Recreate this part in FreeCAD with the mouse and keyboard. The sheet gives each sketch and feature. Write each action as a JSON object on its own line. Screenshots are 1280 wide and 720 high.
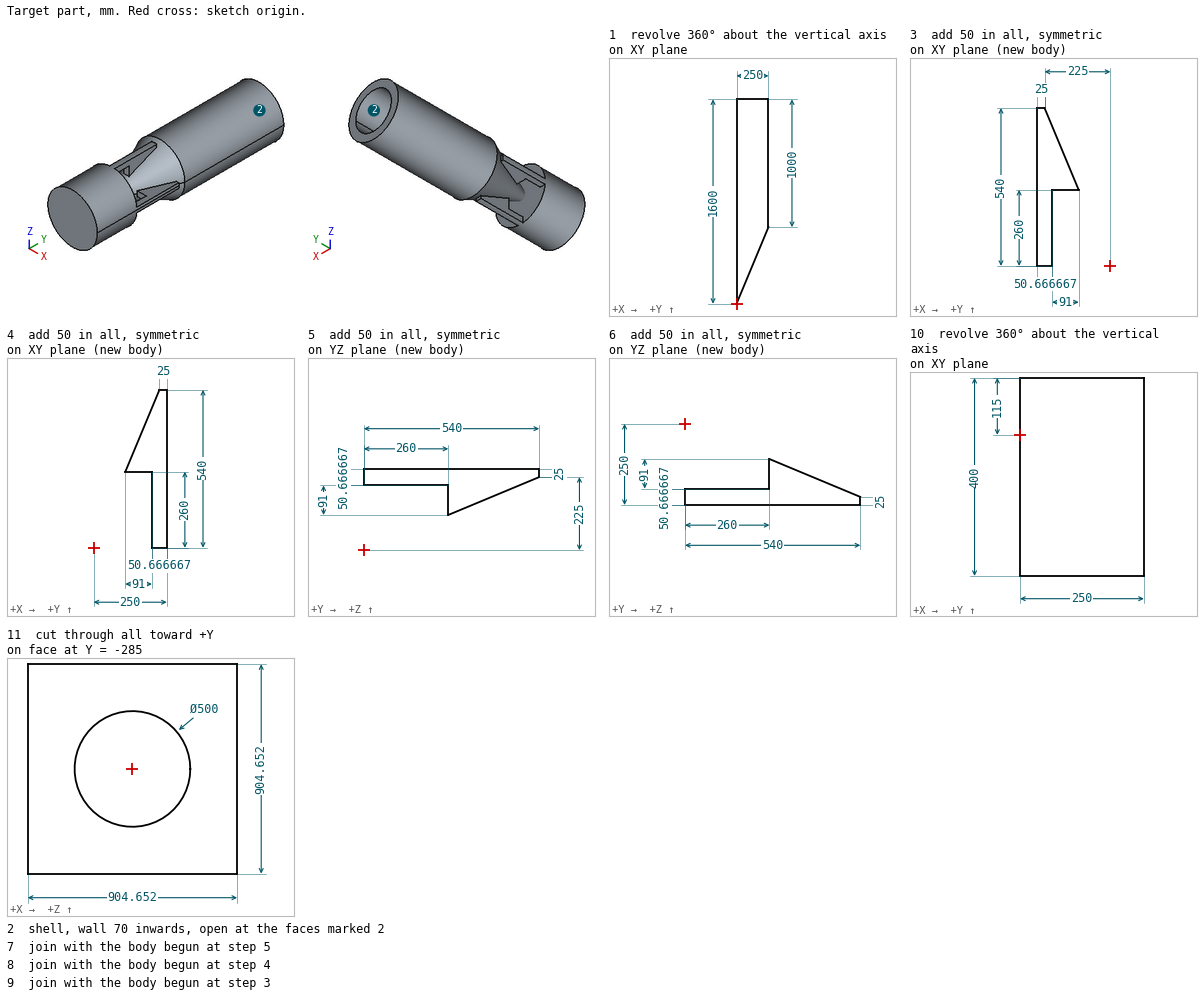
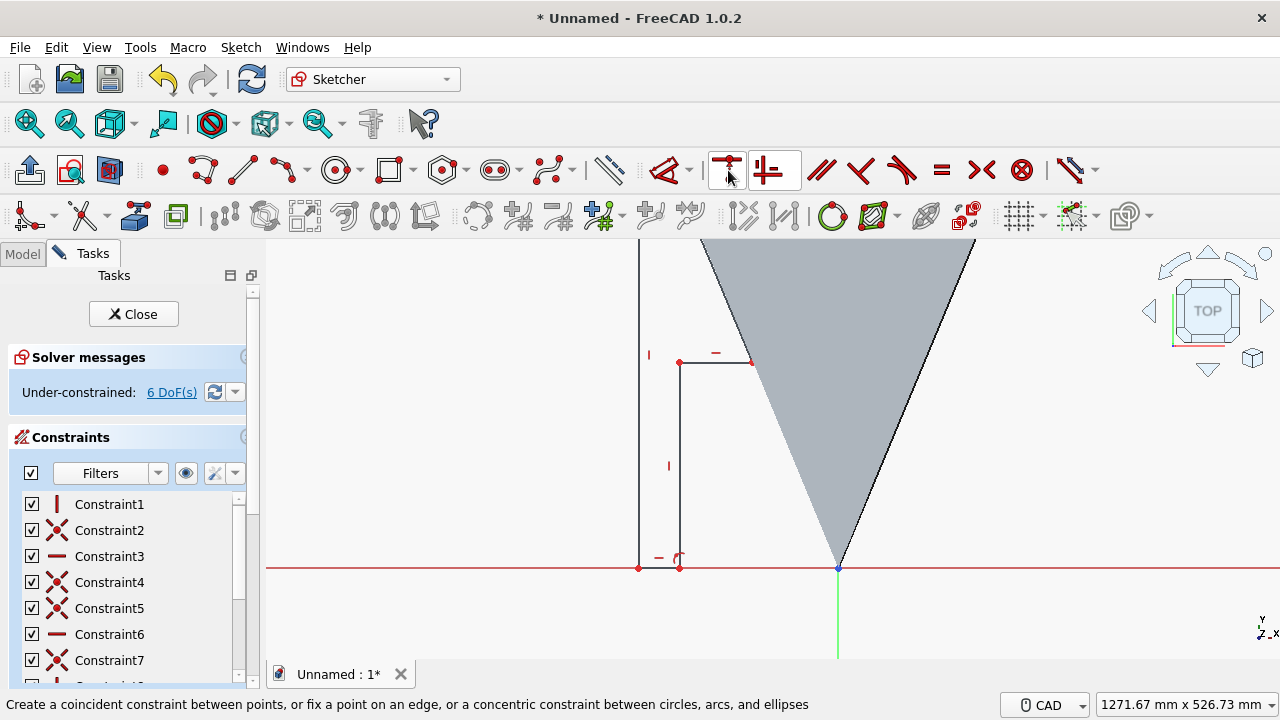
{"action": "left_click", "coordinate": [664, 170]}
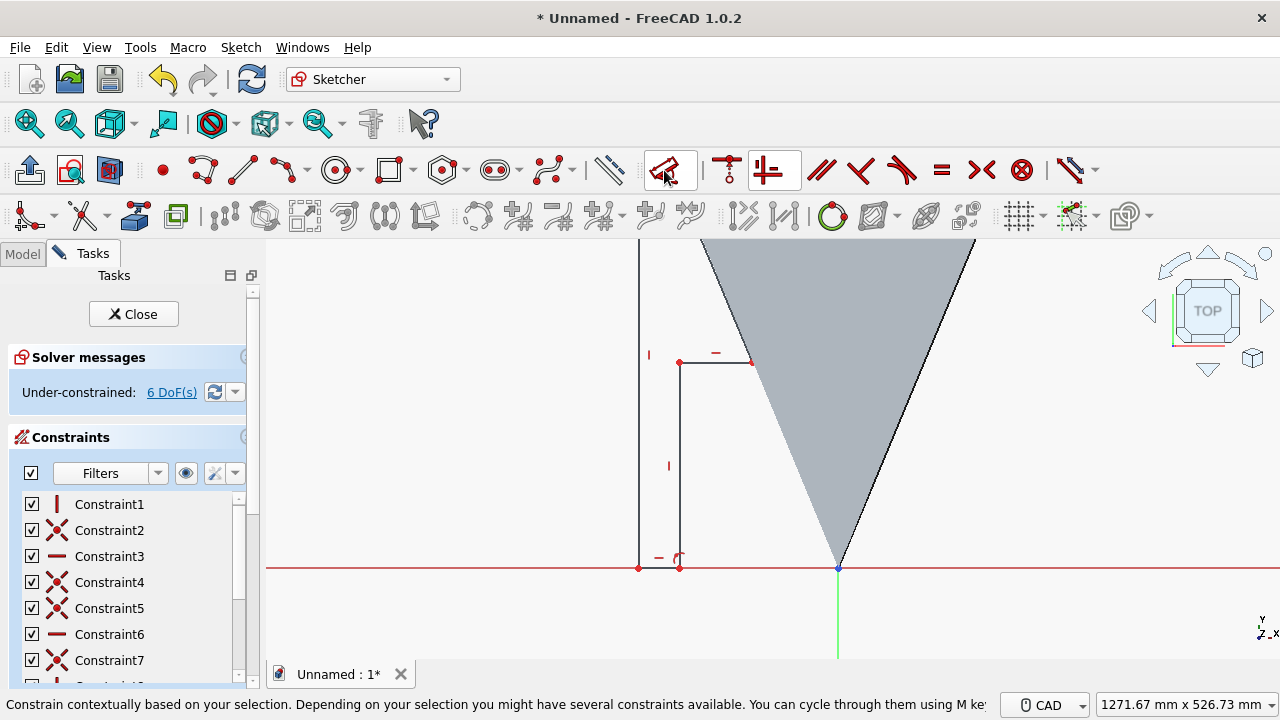
{"action": "left_click", "coordinate": [702, 363]}
{"action": "left_click", "coordinate": [716, 397]}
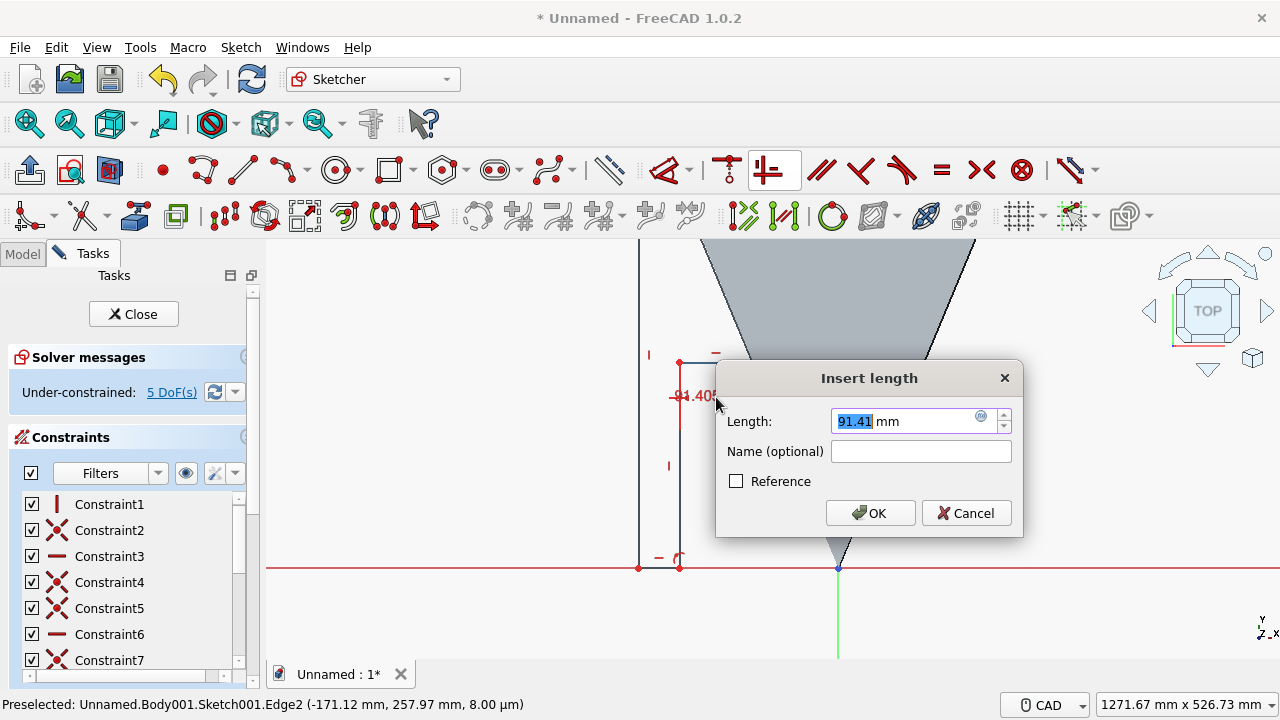
{"action": "type", "text": "91"}
{"action": "key", "text": "Return"}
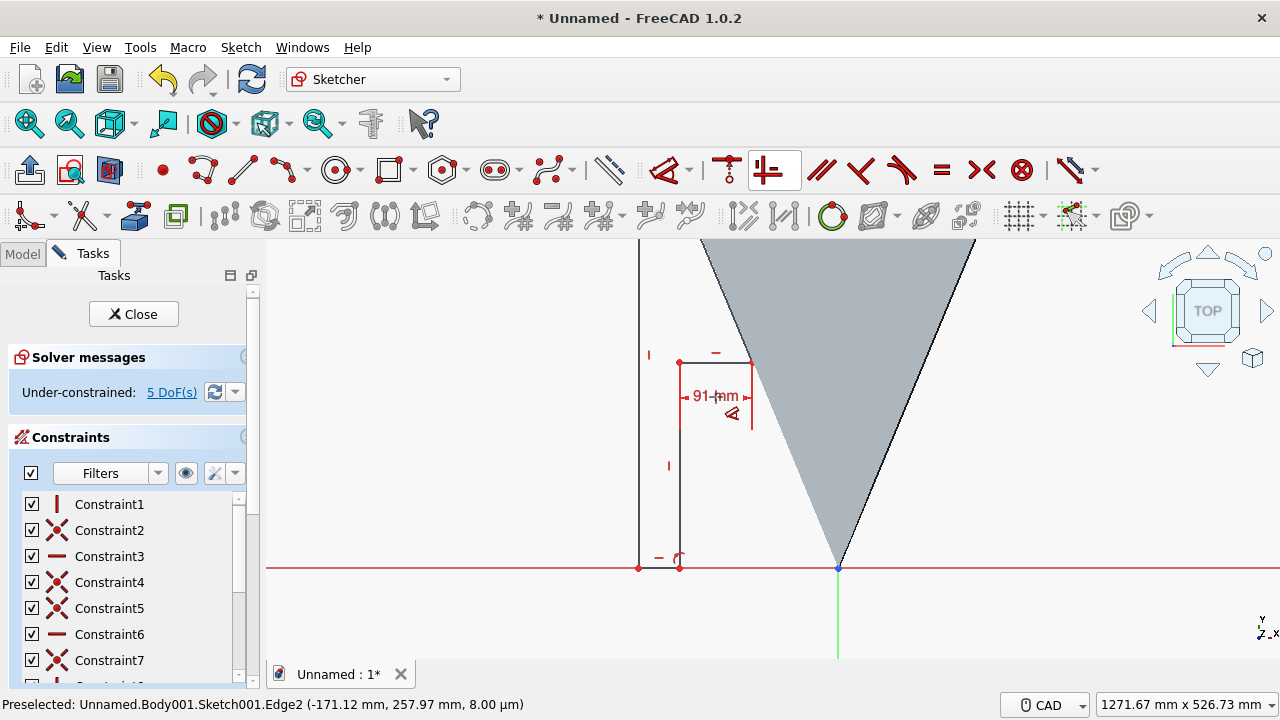
{"action": "scroll", "coordinate": [663, 566], "scroll_direction": "down", "scroll_amount": 3}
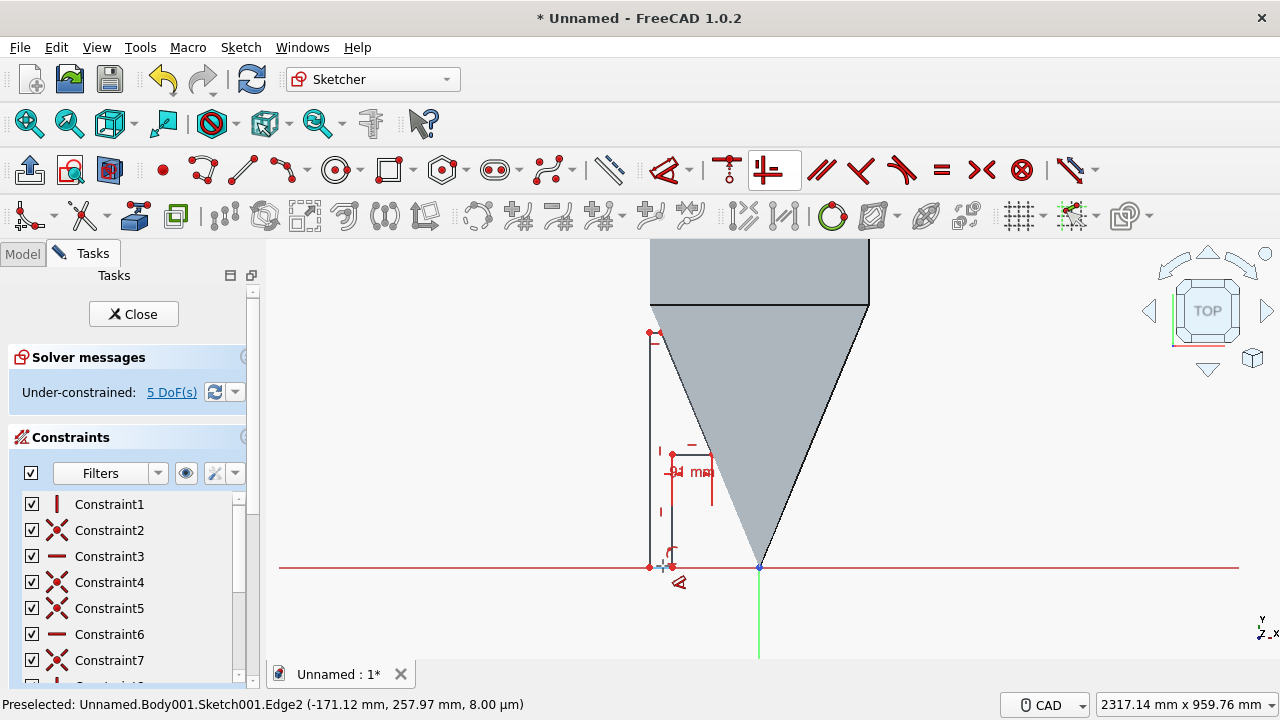
{"action": "scroll", "coordinate": [656, 333], "scroll_direction": "up", "scroll_amount": 7}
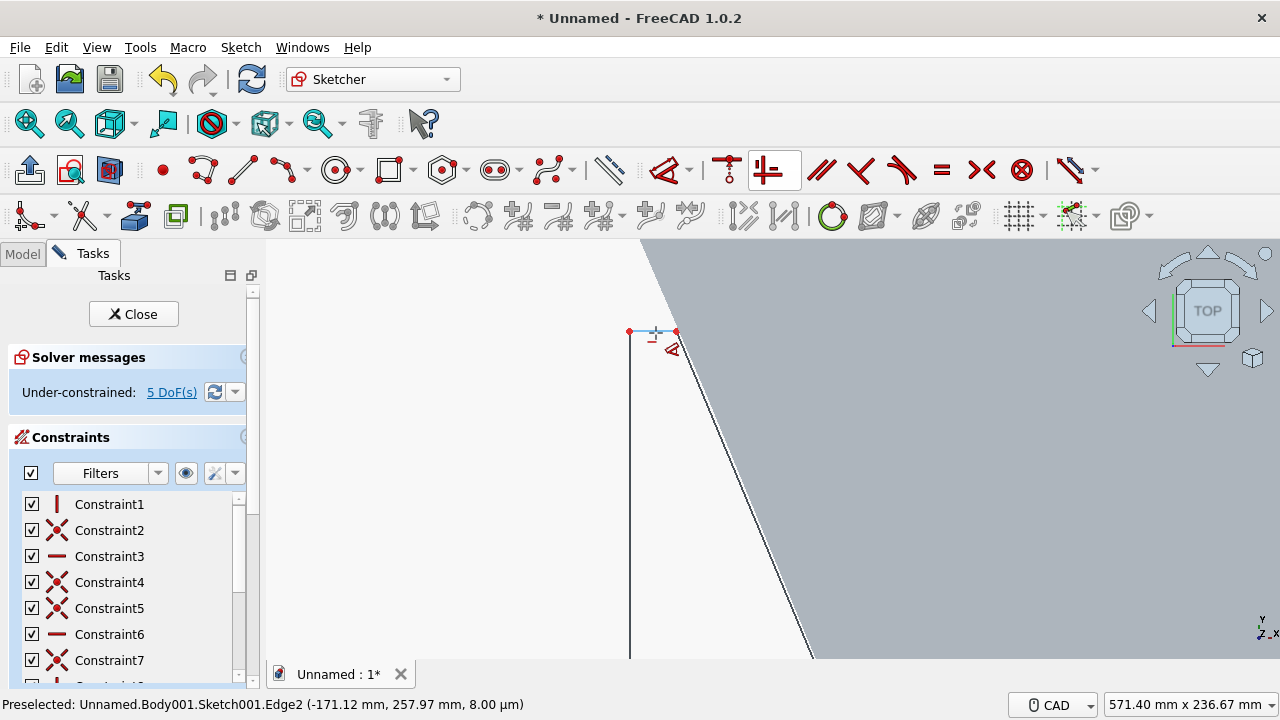
{"action": "left_click", "coordinate": [653, 331]}
{"action": "left_click", "coordinate": [653, 297]}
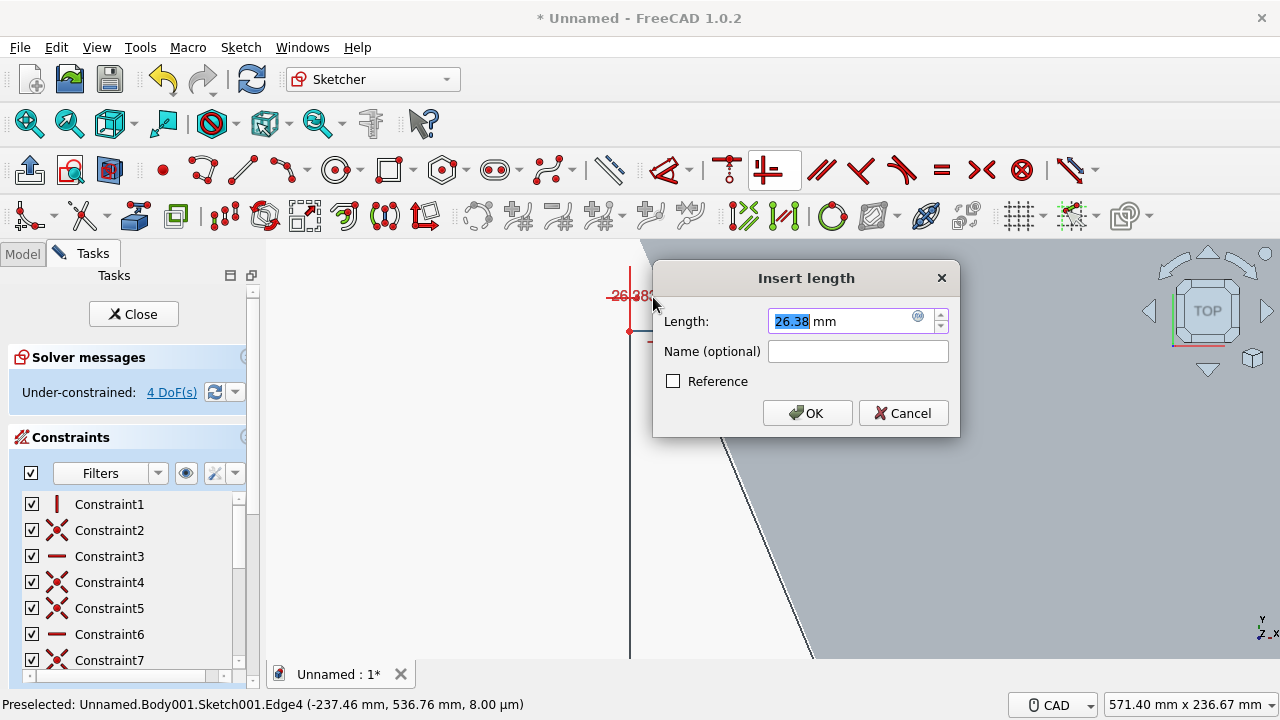
{"action": "type", "text": "25"}
{"action": "key", "text": "Return"}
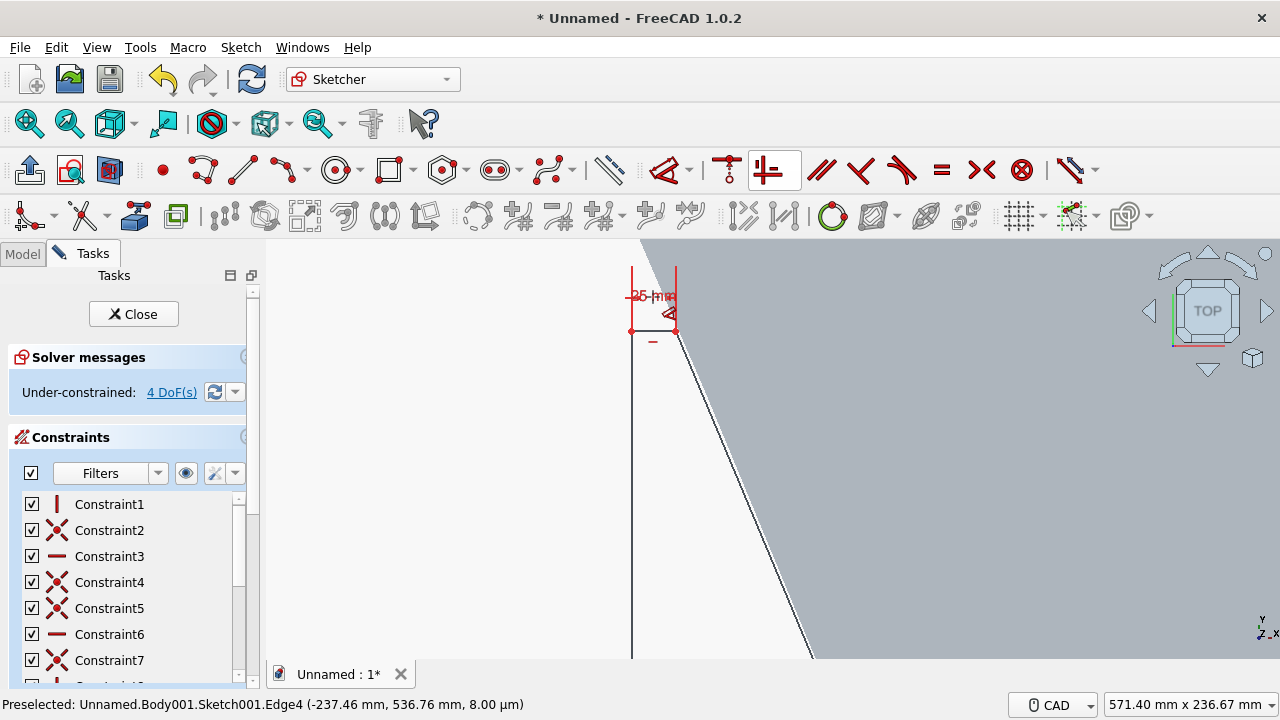
{"action": "scroll", "coordinate": [656, 333], "scroll_direction": "down", "scroll_amount": 7}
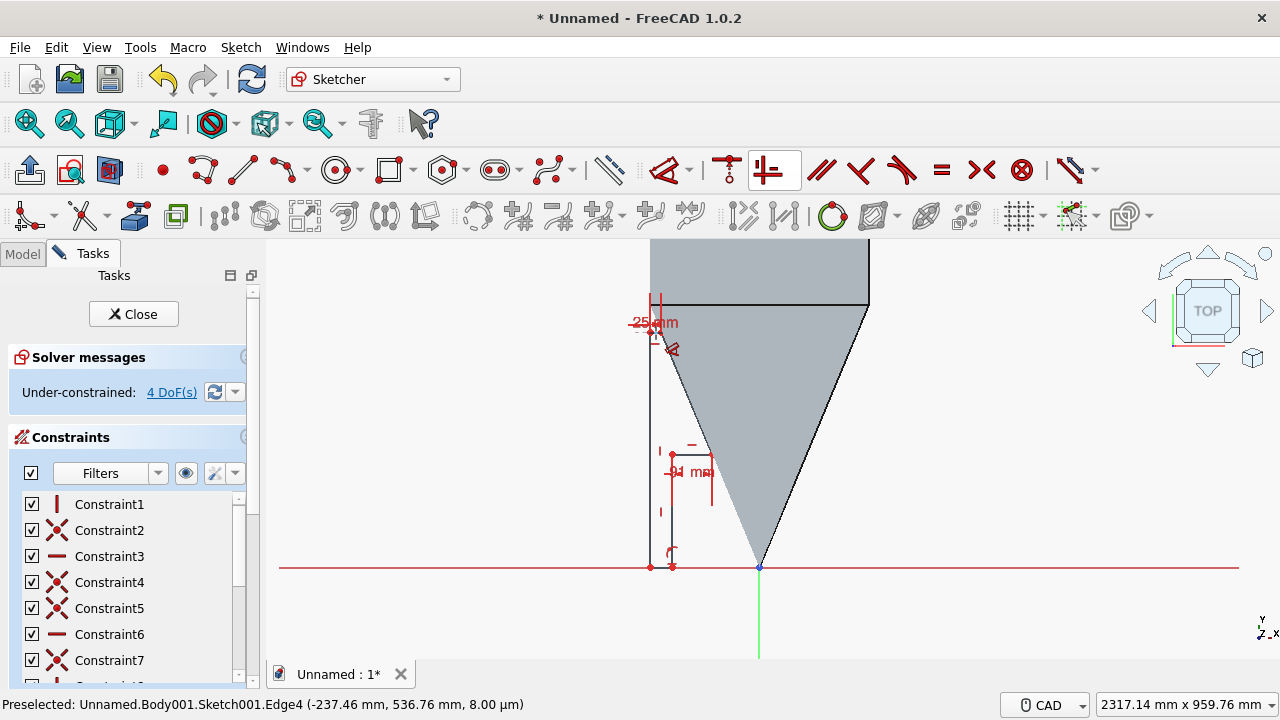
{"action": "left_click", "coordinate": [672, 534]}
{"action": "left_click", "coordinate": [706, 511]}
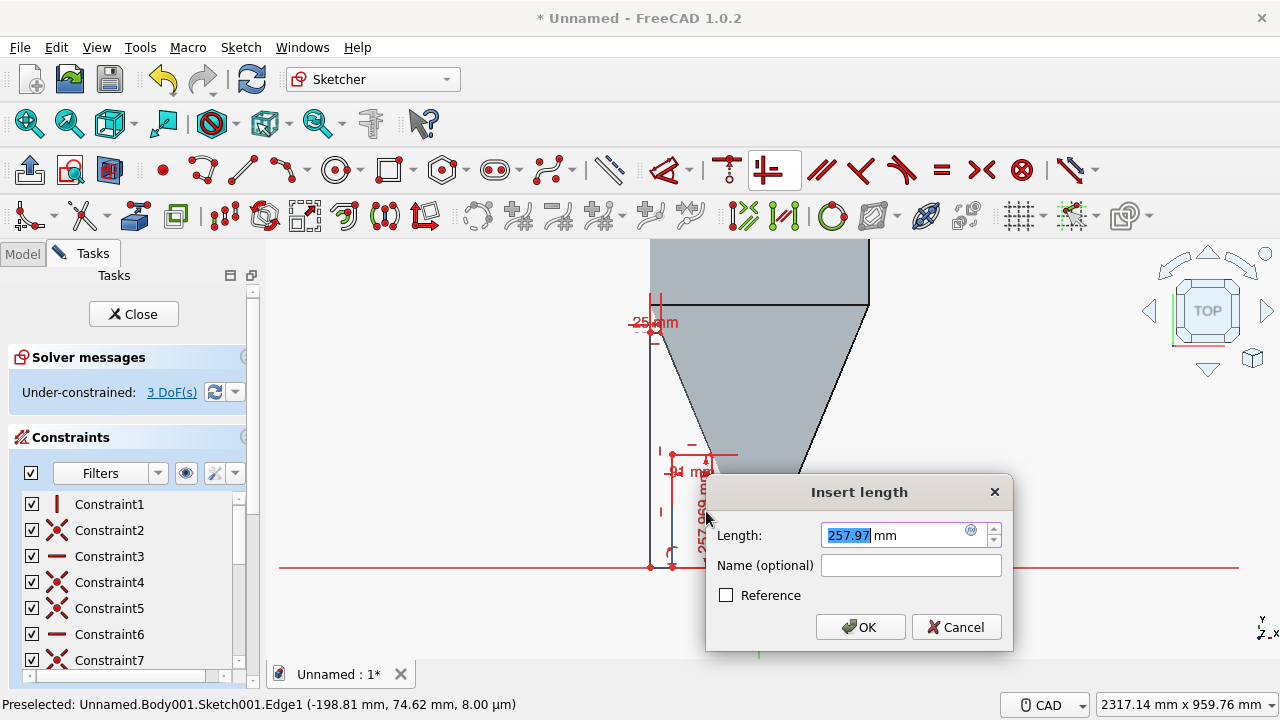
{"action": "type", "text": "260"}
{"action": "key", "text": "Return"}